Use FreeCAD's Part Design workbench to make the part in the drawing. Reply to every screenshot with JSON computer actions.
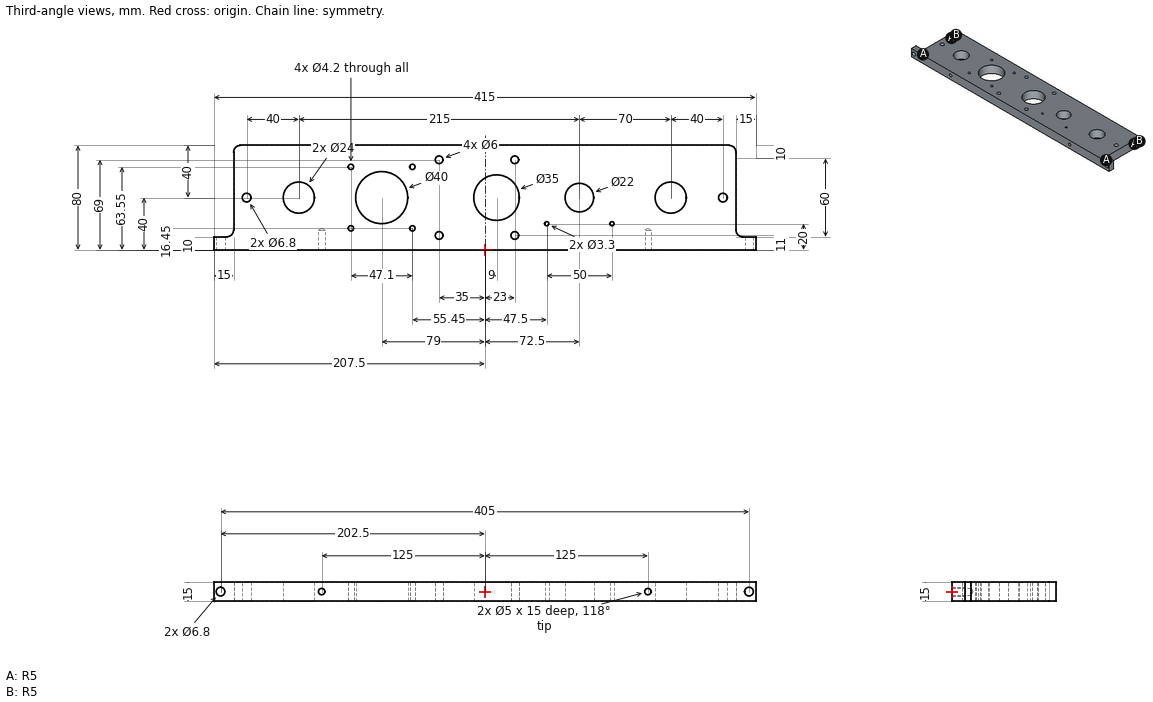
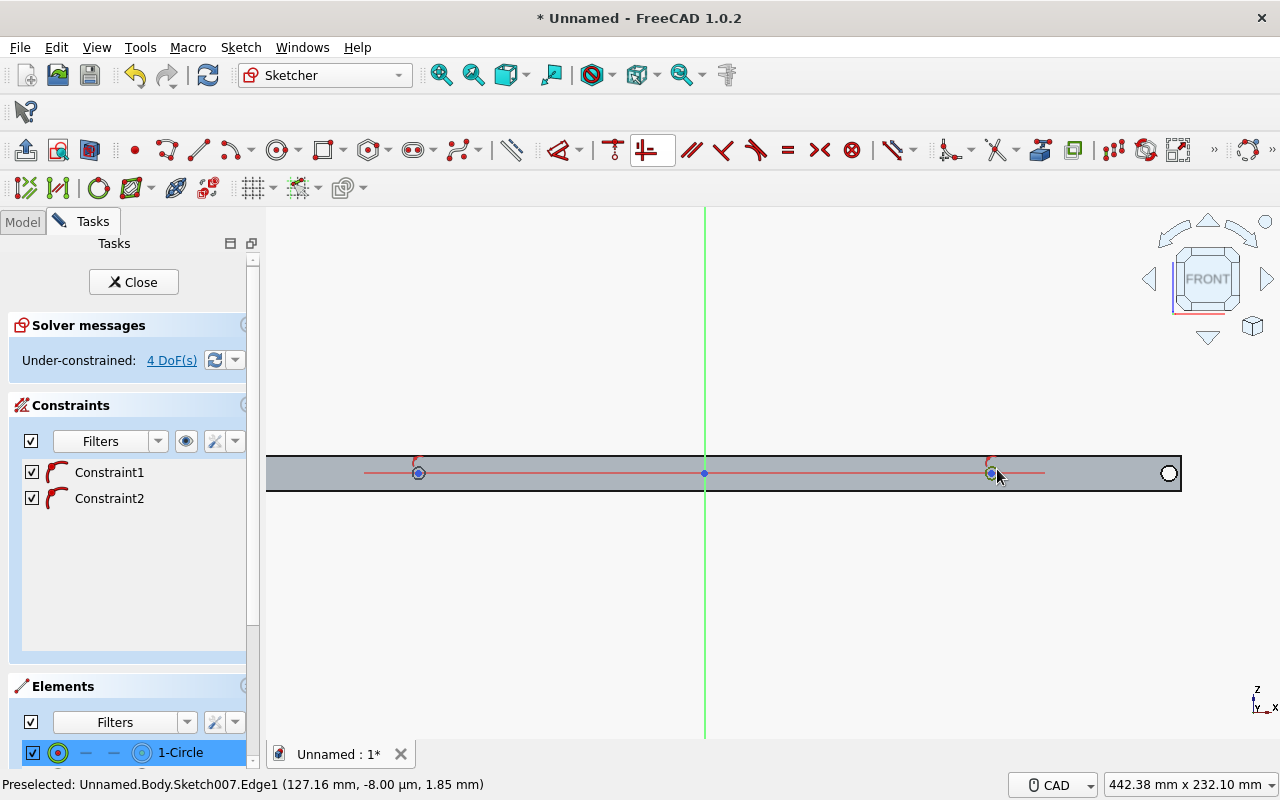
{"action": "scroll", "coordinate": [423, 469], "scroll_direction": "up", "scroll_amount": 6}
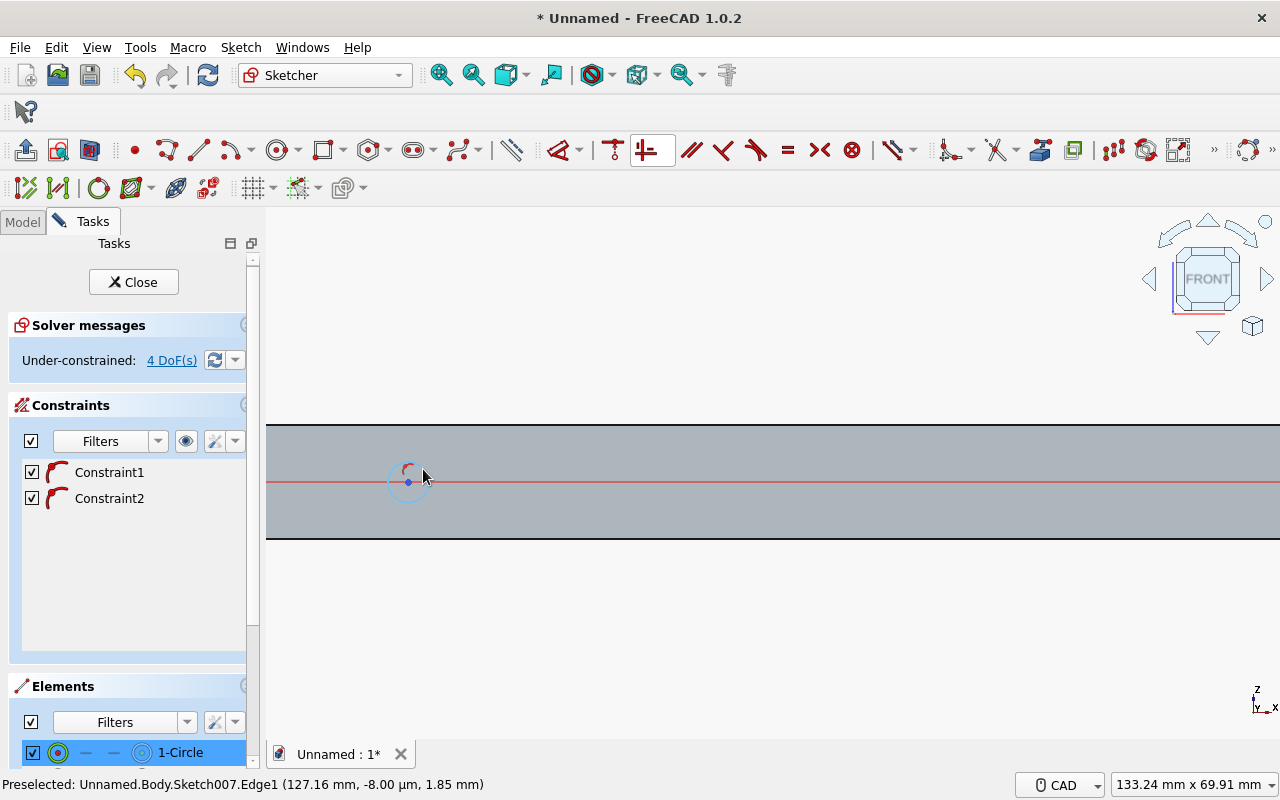
{"action": "left_click", "coordinate": [423, 468]}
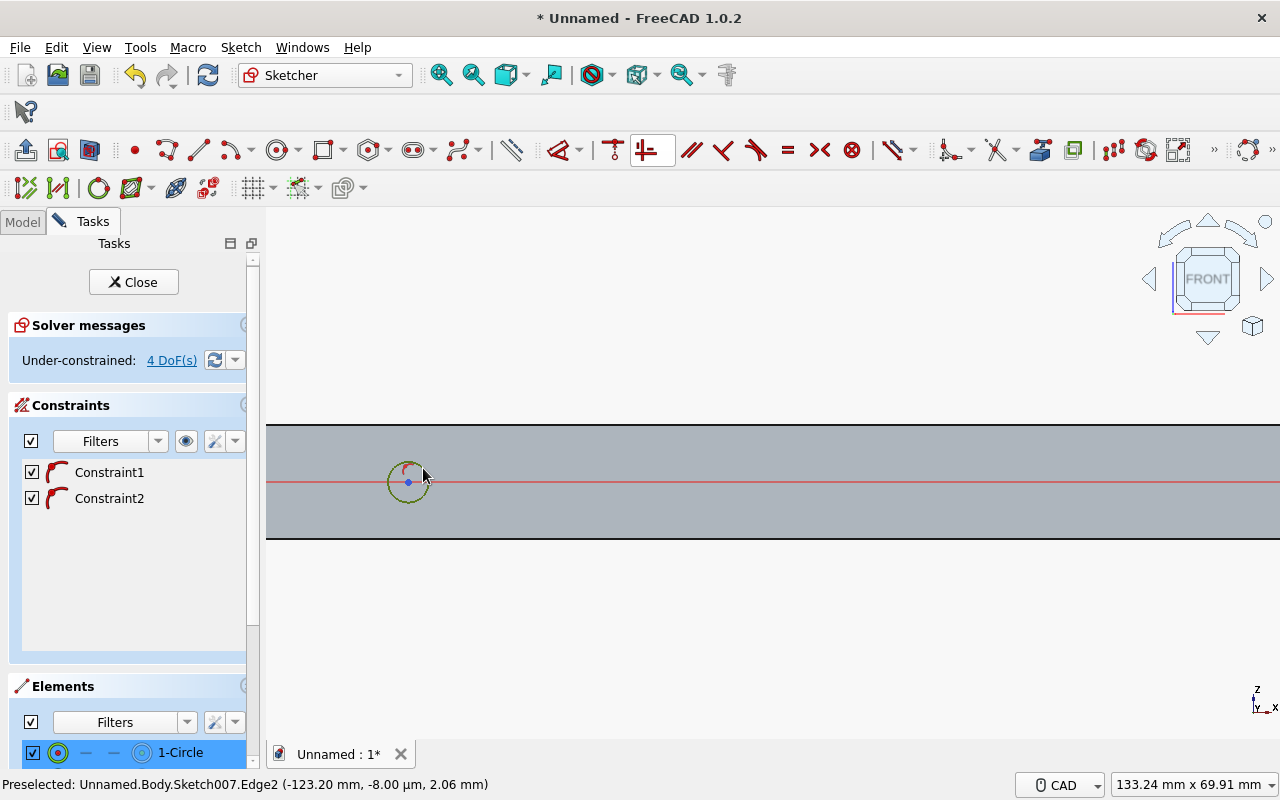
{"action": "left_click", "coordinate": [788, 150]}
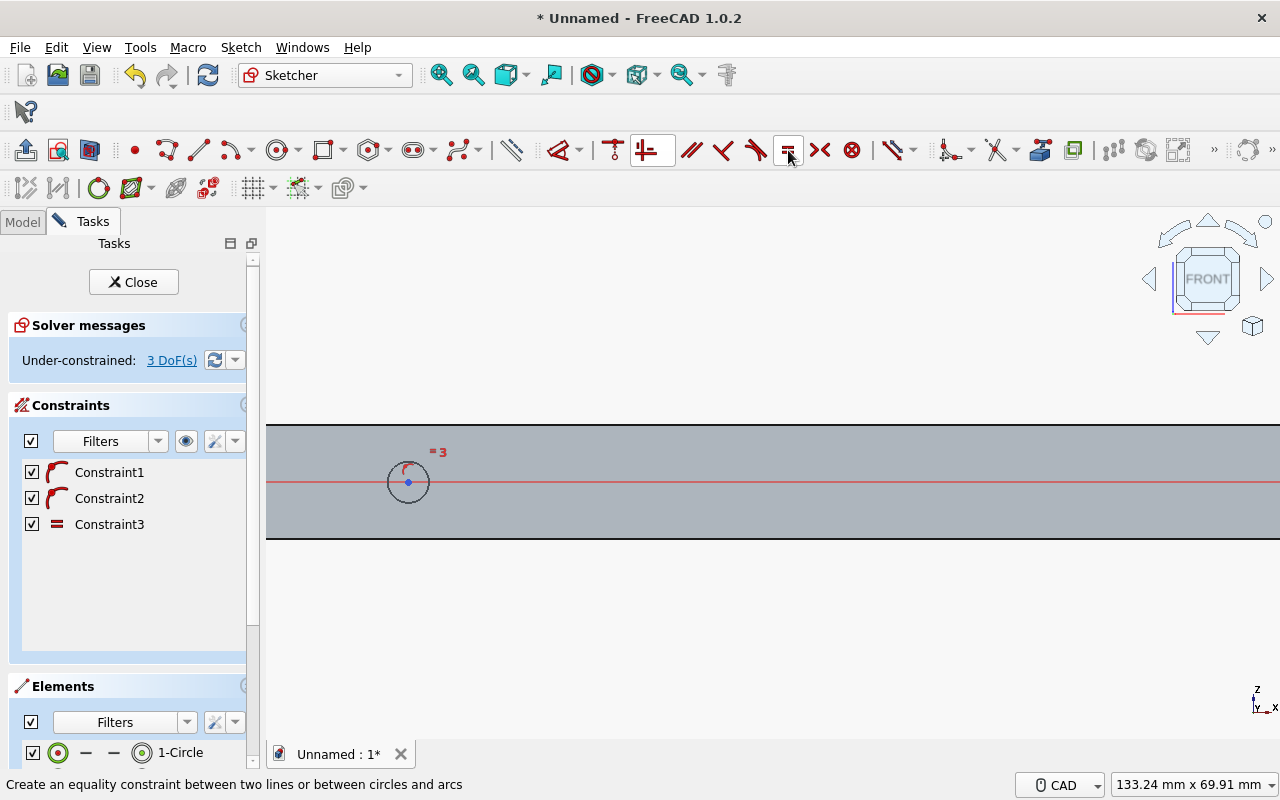
{"action": "left_click", "coordinate": [558, 150]}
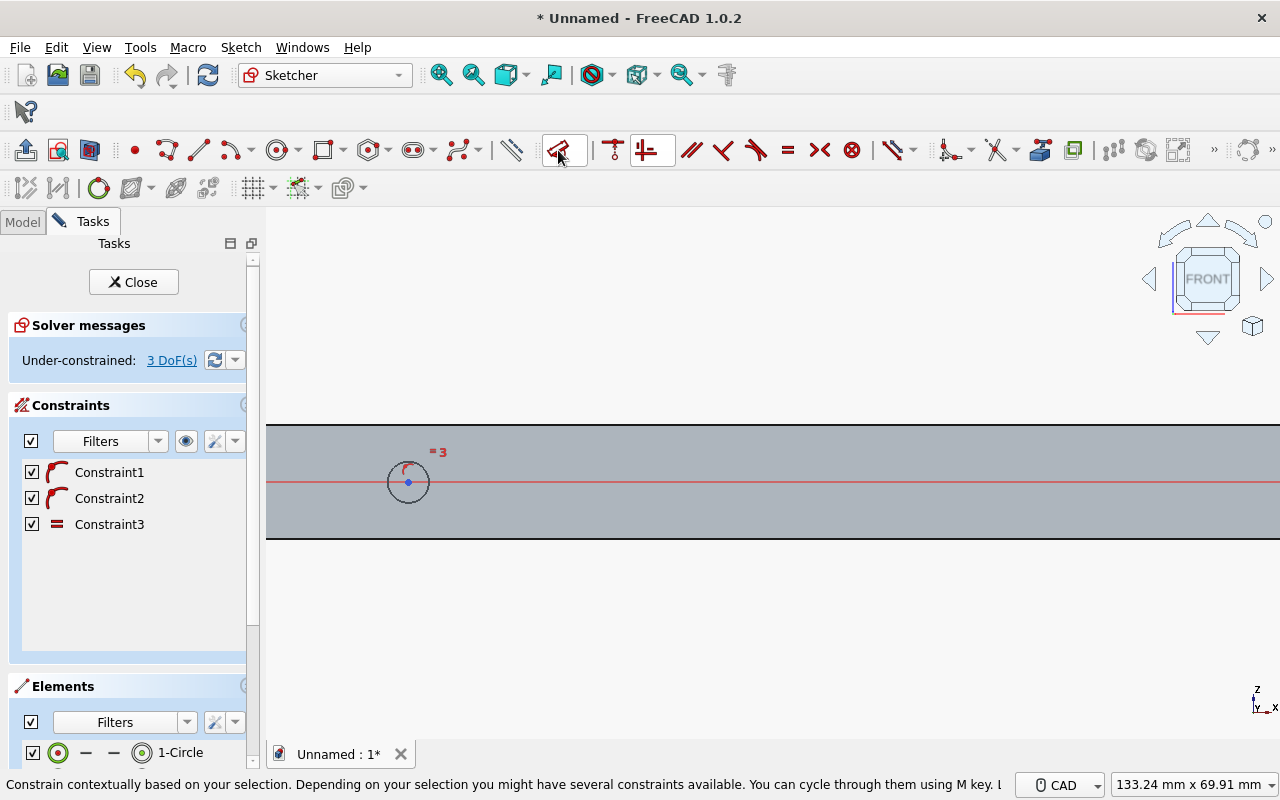
{"action": "scroll", "coordinate": [422, 469], "scroll_direction": "down", "scroll_amount": 6}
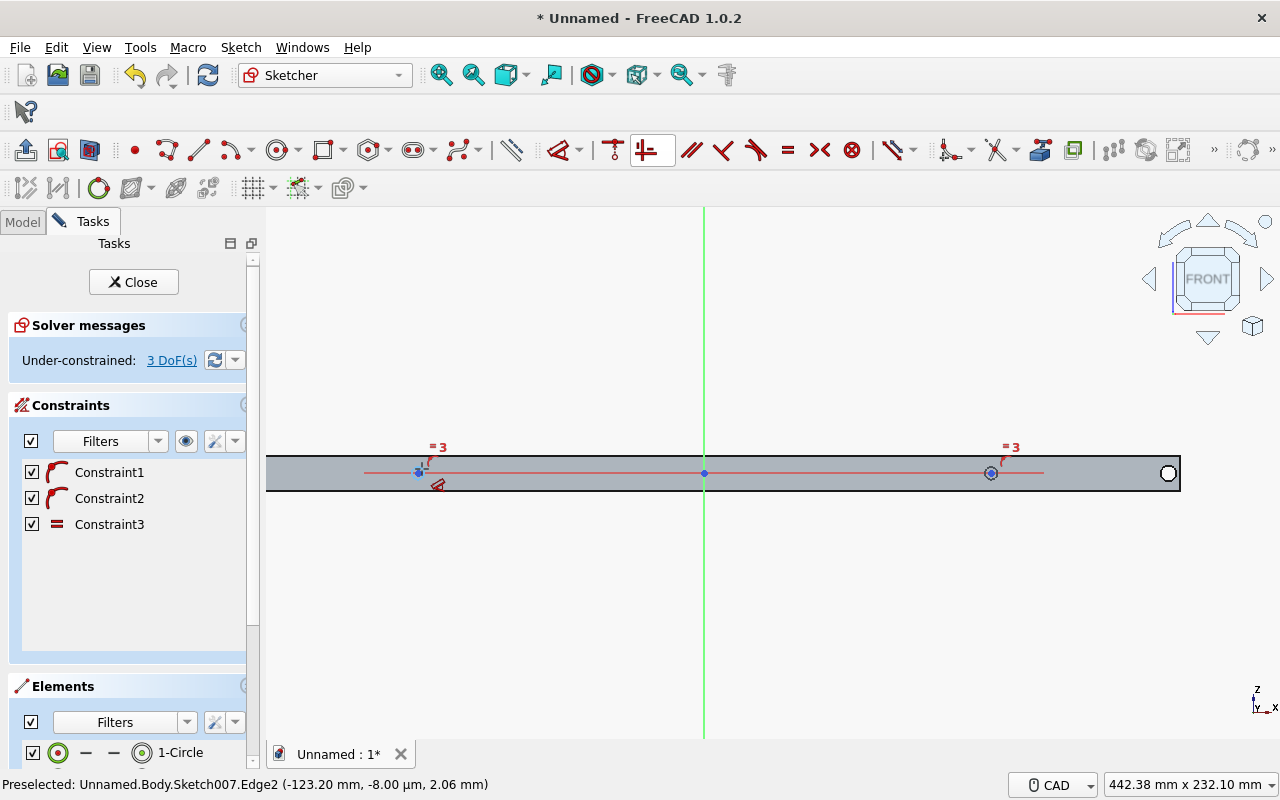
{"action": "scroll", "coordinate": [996, 469], "scroll_direction": "up", "scroll_amount": 7}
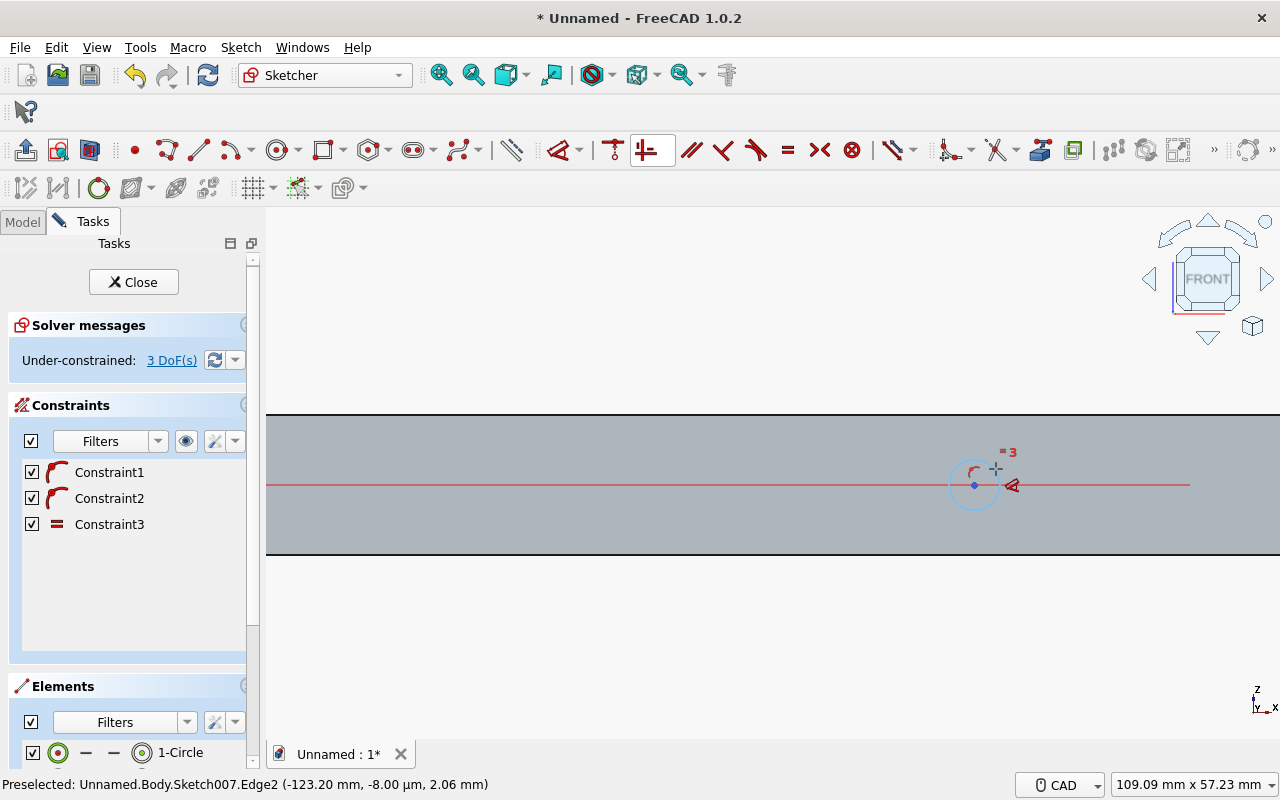
{"action": "left_click", "coordinate": [992, 467]}
{"action": "left_click", "coordinate": [1014, 444]}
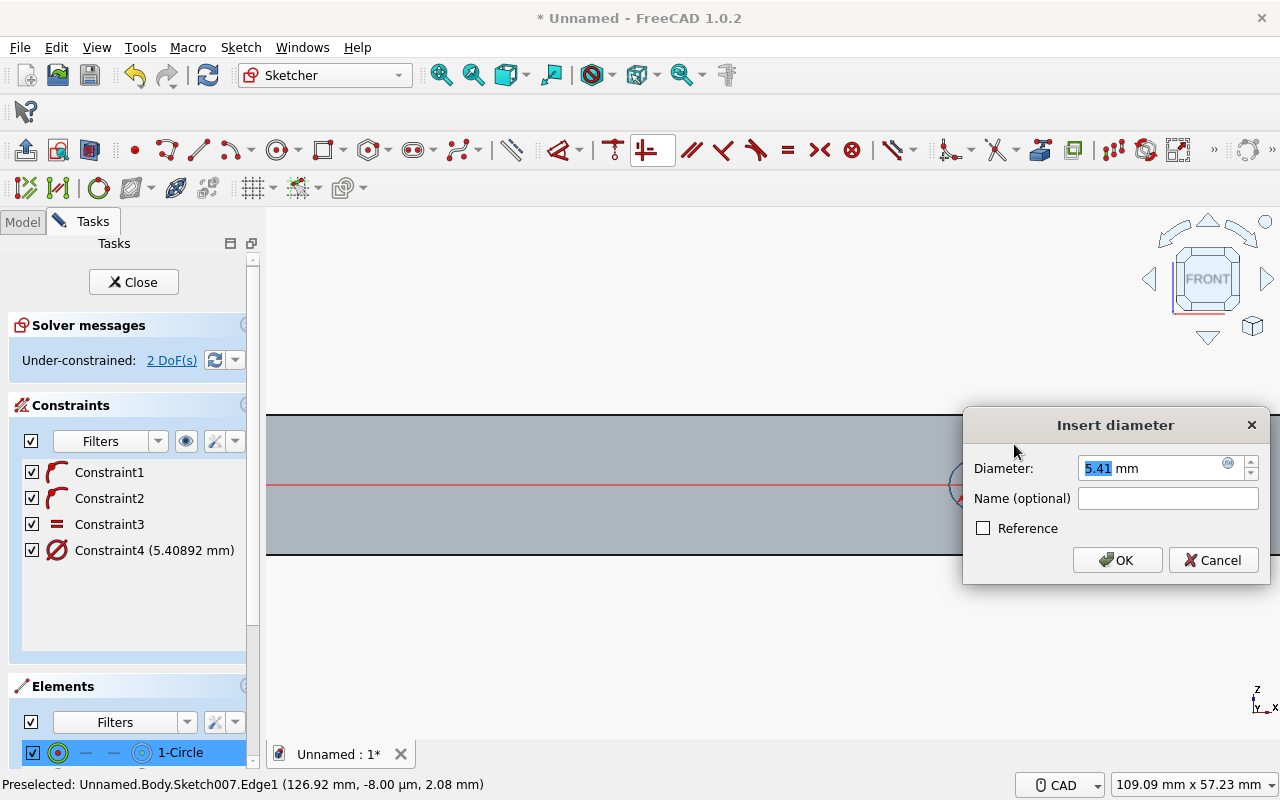
{"action": "type", "text": "5"}
{"action": "key", "text": "Return"}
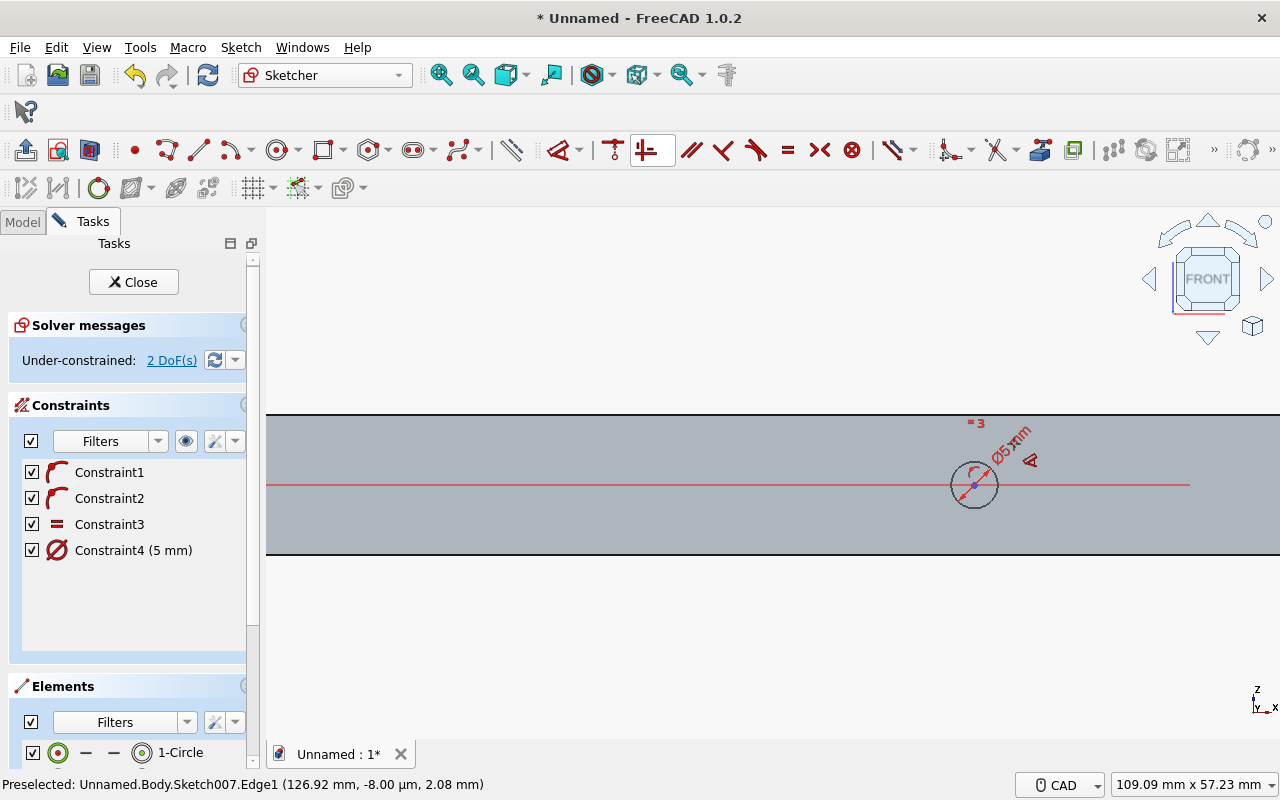
{"action": "scroll", "coordinate": [997, 469], "scroll_direction": "down", "scroll_amount": 7}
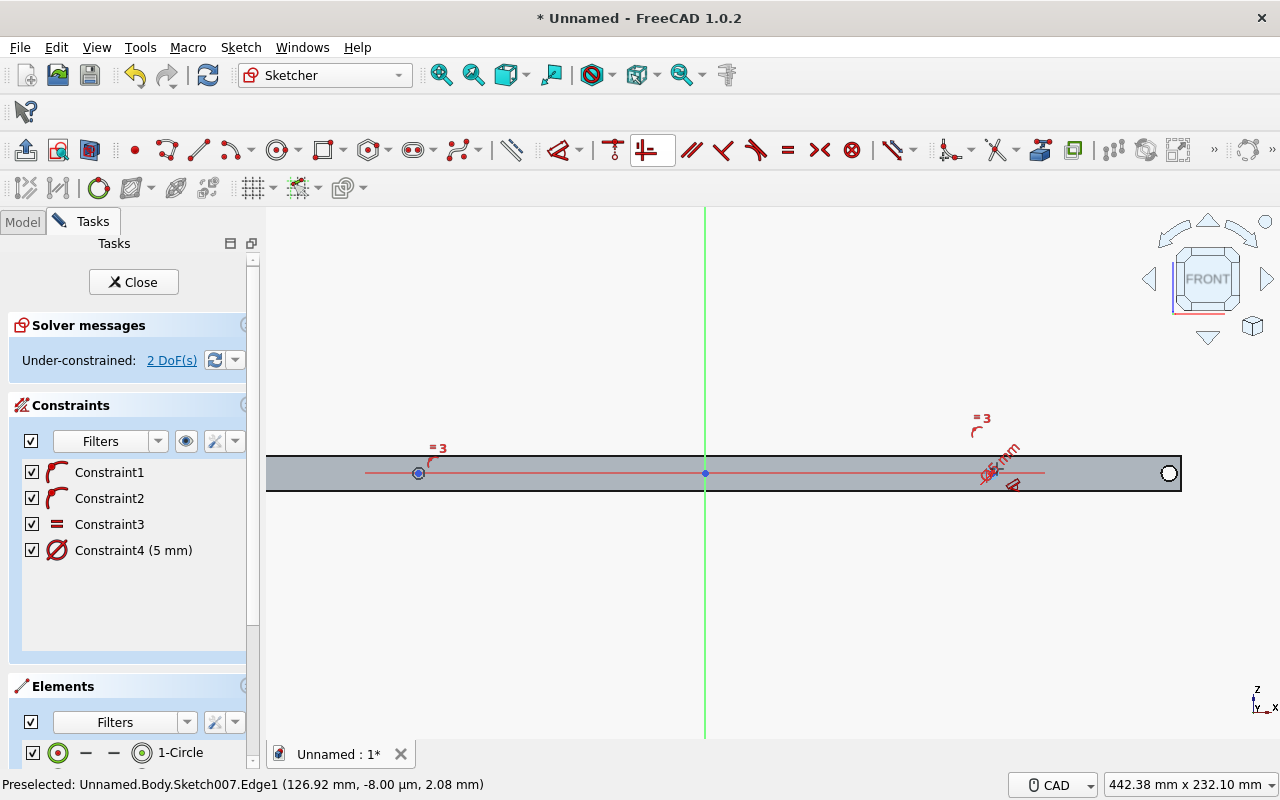
{"action": "left_click", "coordinate": [992, 473]}
{"action": "left_click", "coordinate": [849, 507]}